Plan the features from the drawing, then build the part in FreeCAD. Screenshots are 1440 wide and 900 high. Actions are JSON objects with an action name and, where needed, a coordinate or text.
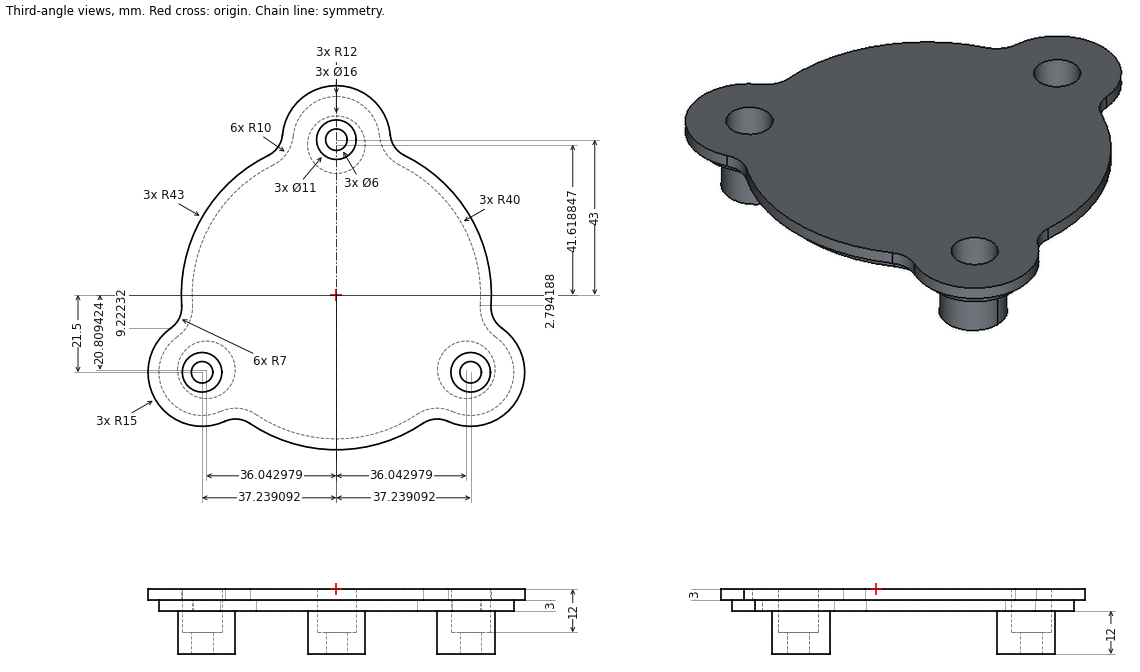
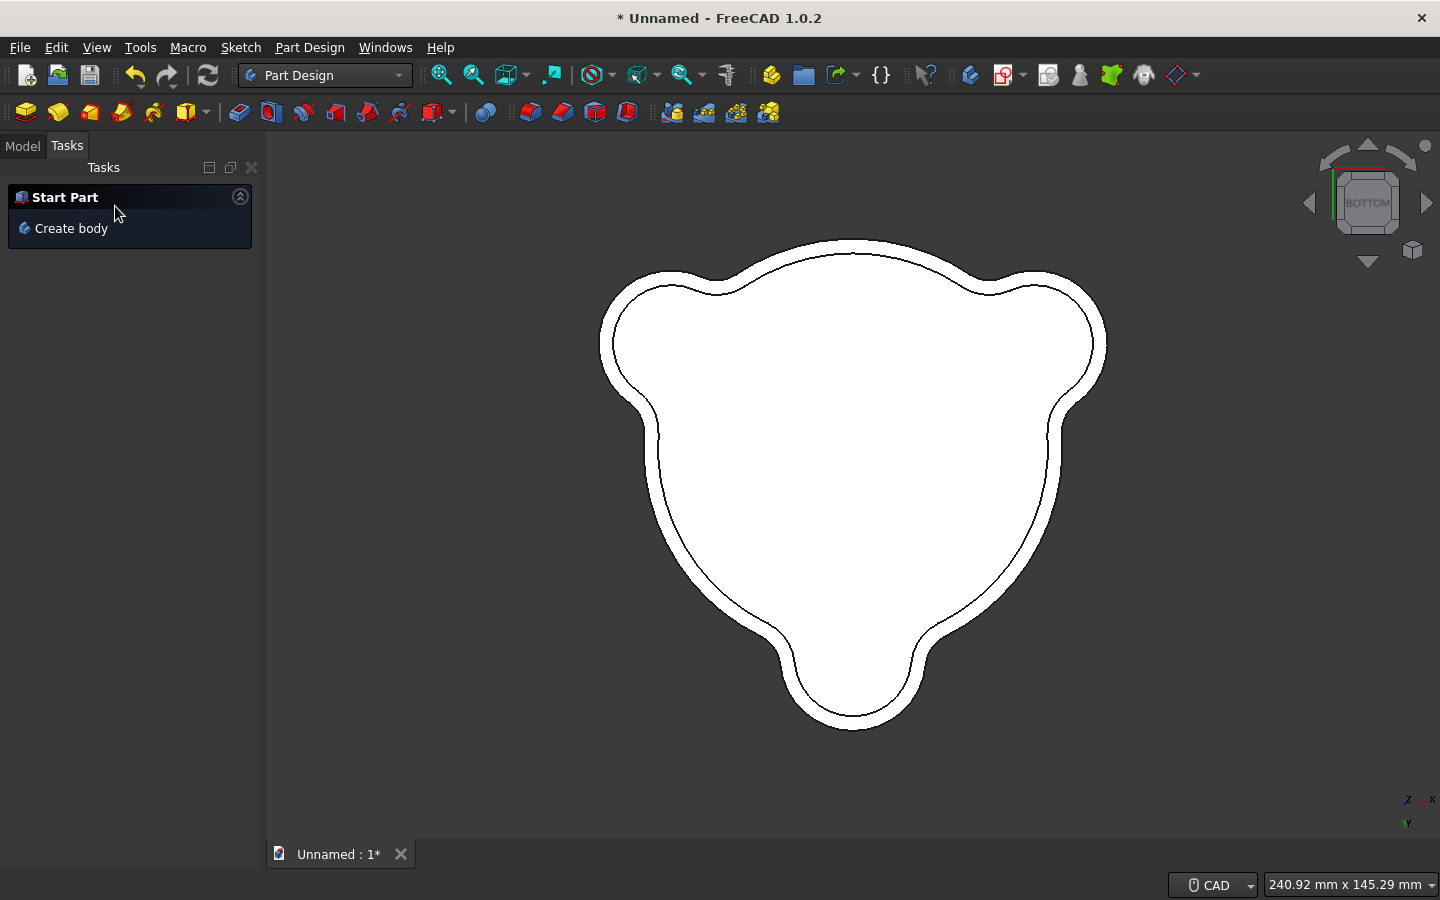
{"action": "left_click", "coordinate": [853, 418]}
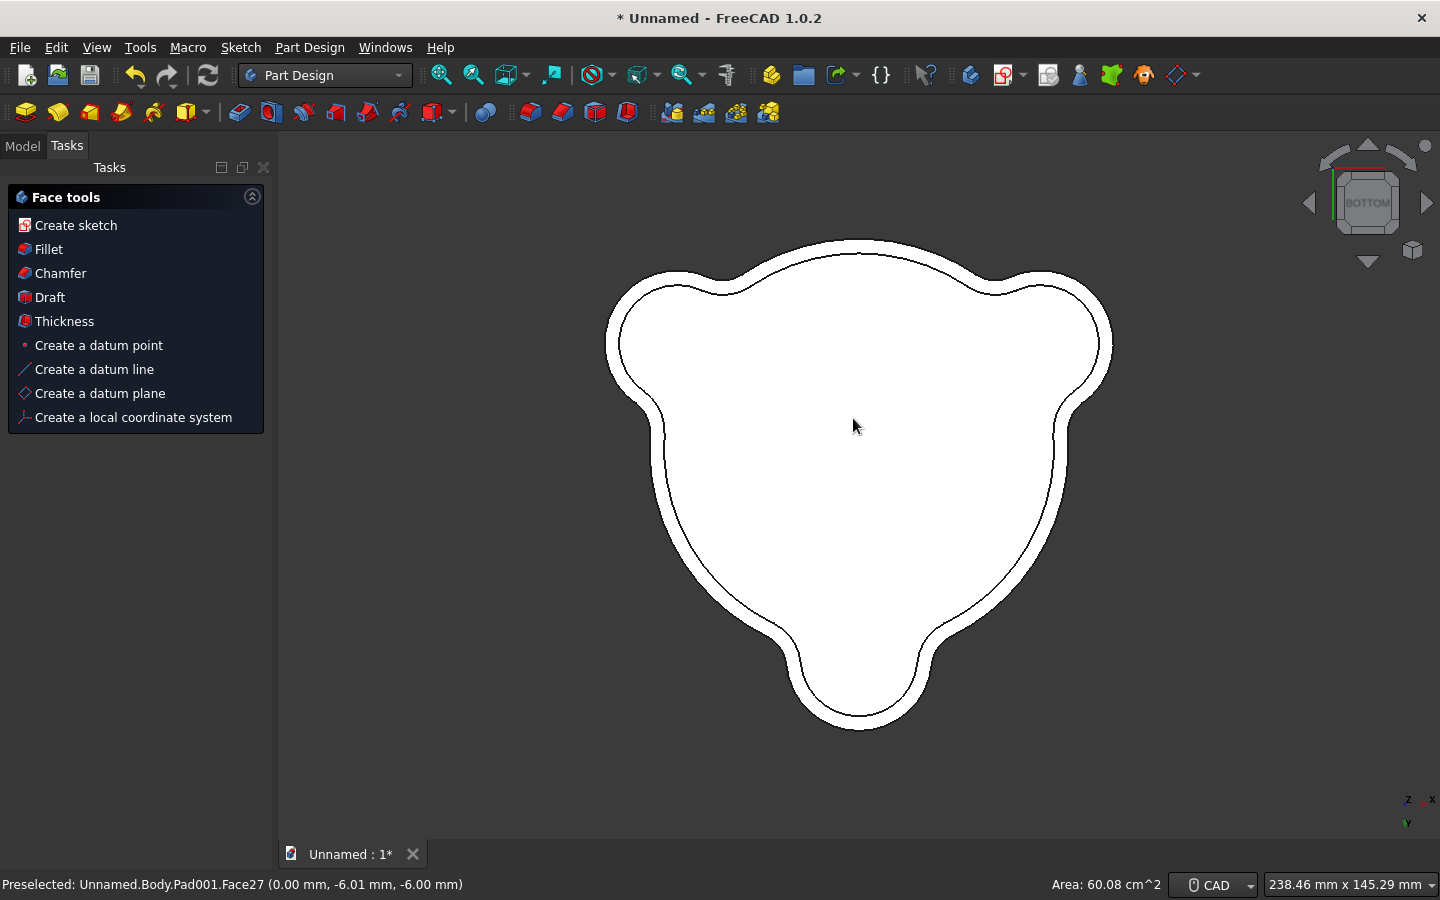
{"action": "left_click", "coordinate": [1004, 76]}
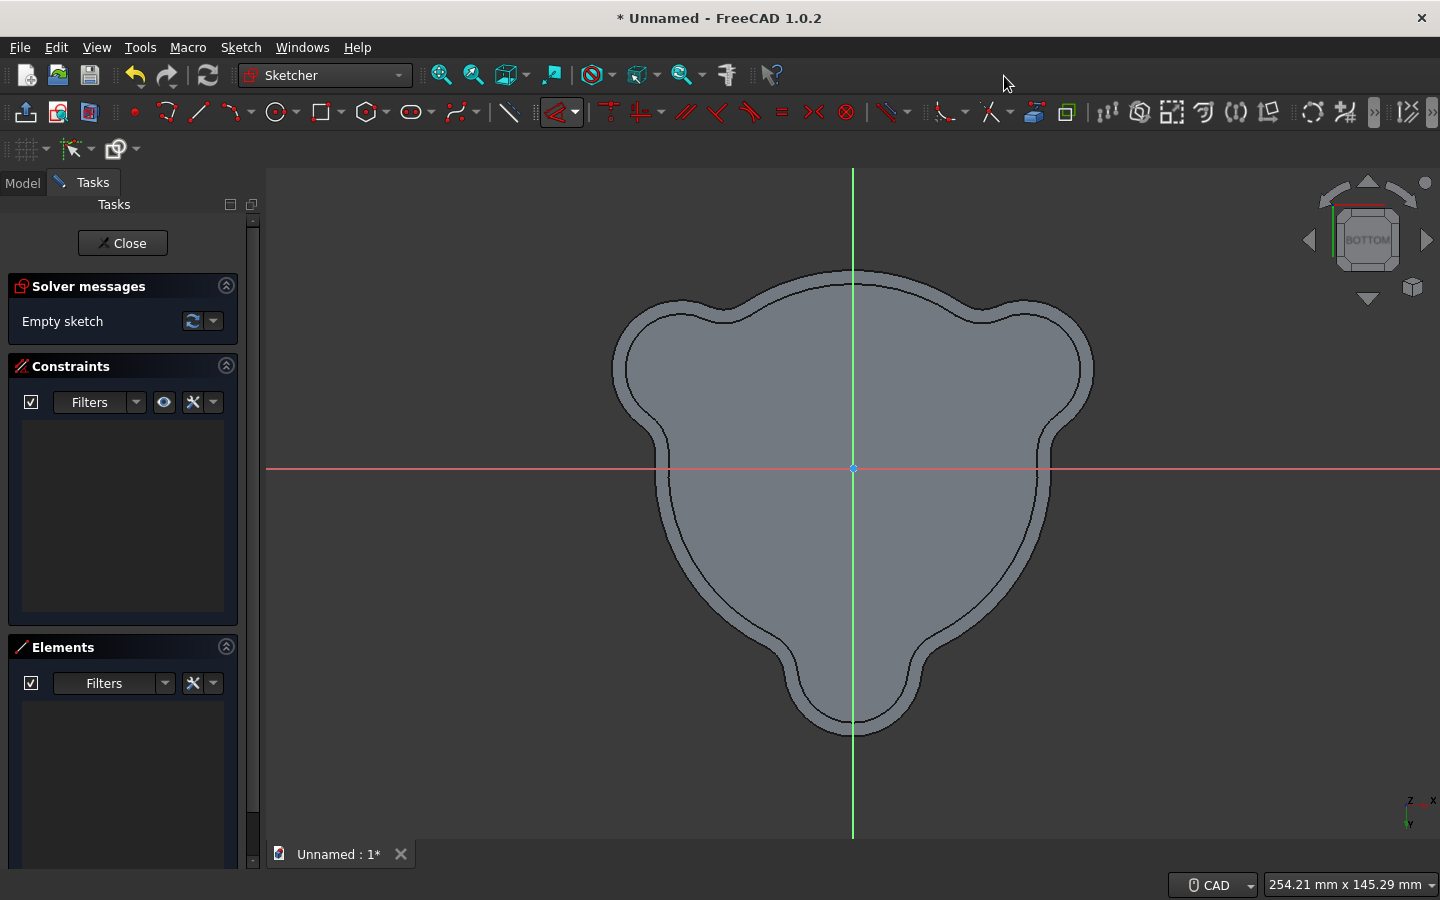
{"action": "left_click", "coordinate": [276, 112]}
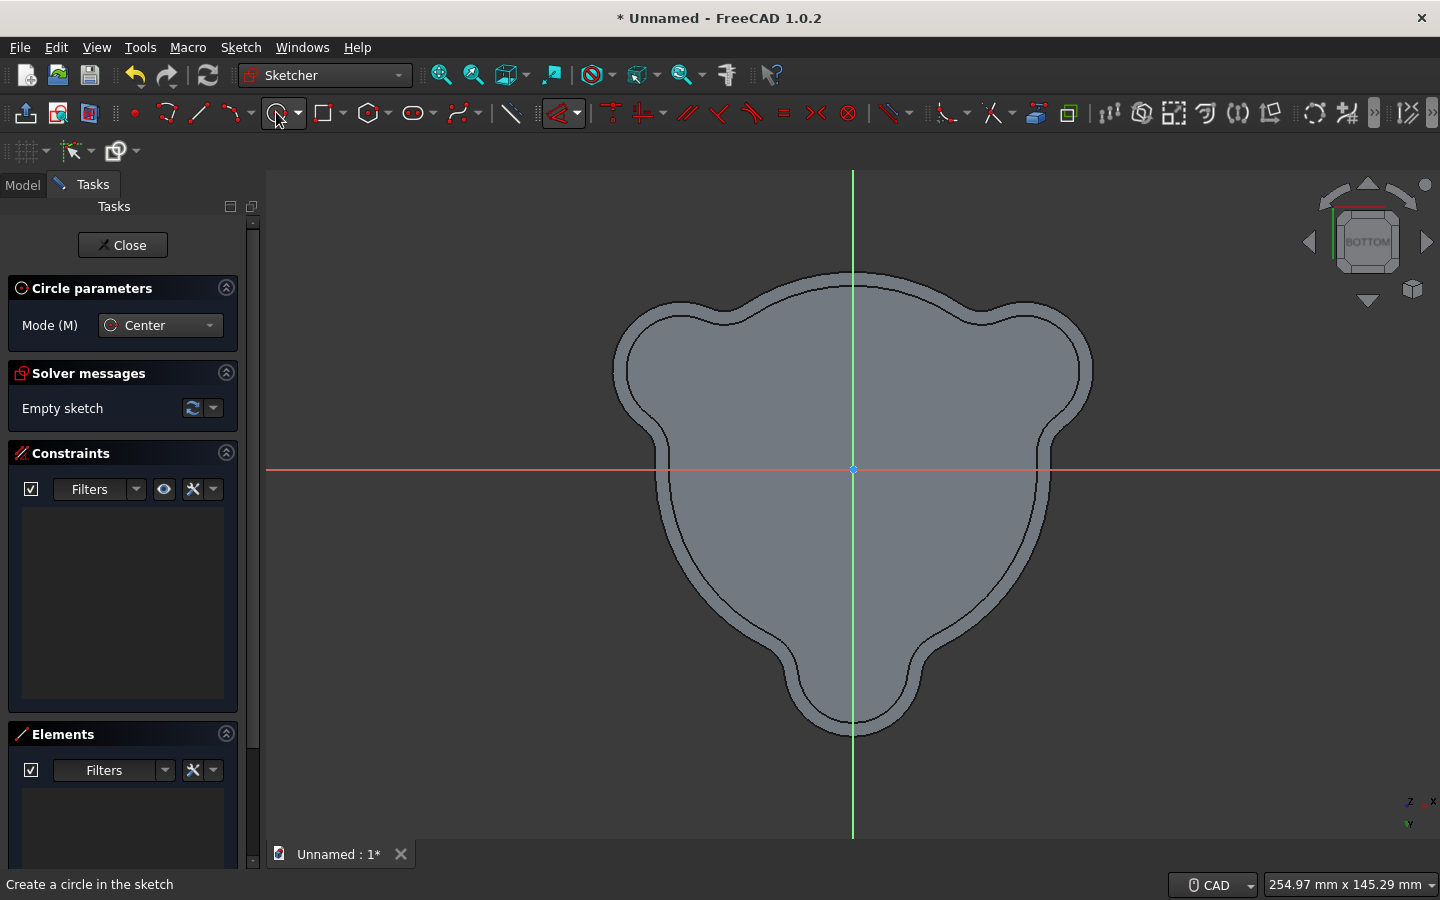
{"action": "left_click", "coordinate": [853, 661]}
{"action": "left_click", "coordinate": [879, 635]}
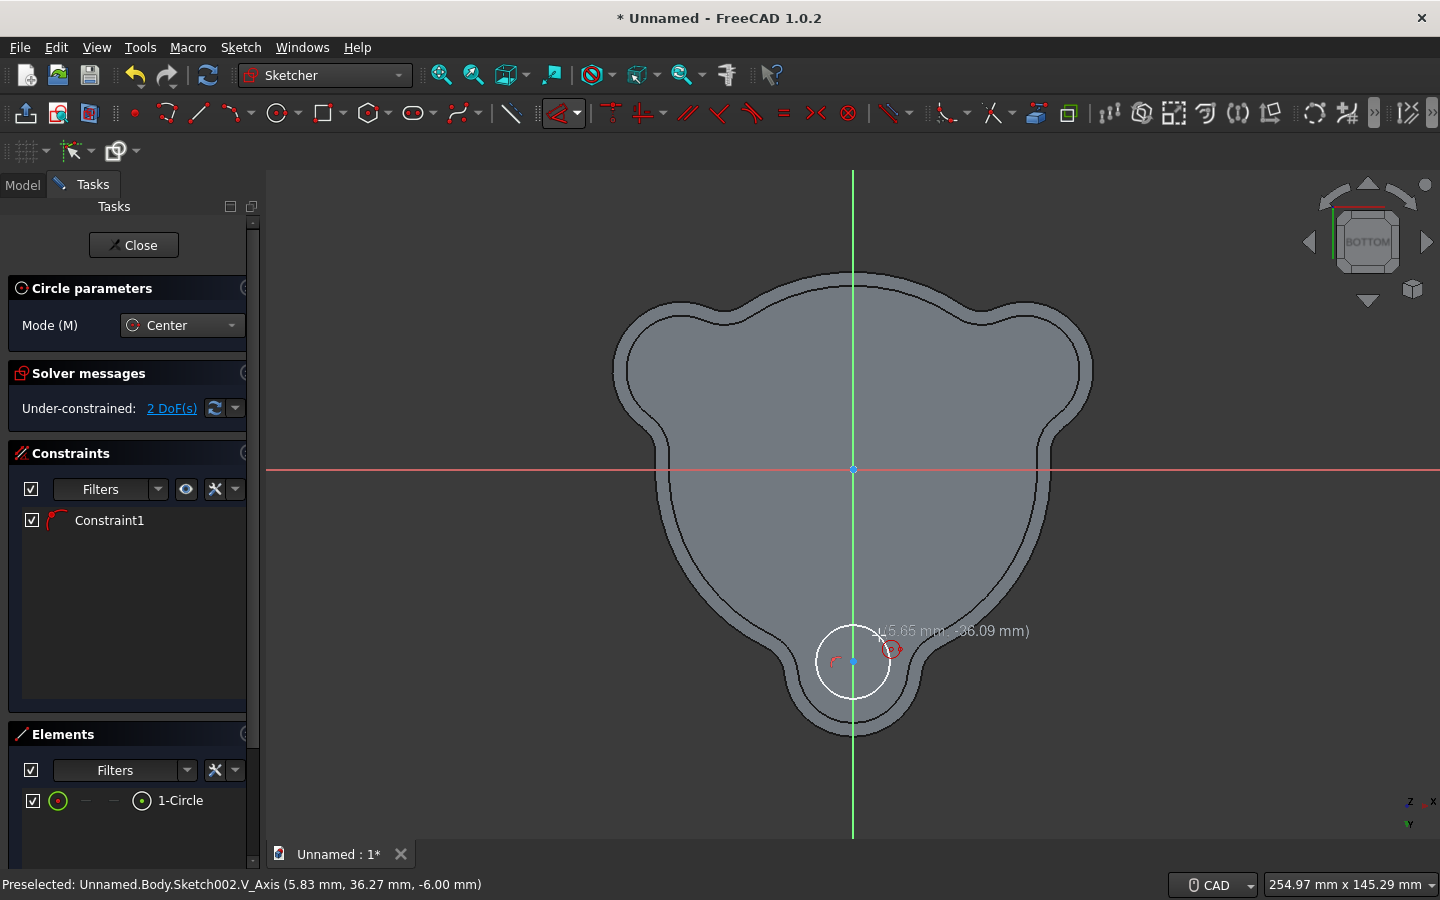
{"action": "left_click", "coordinate": [687, 374]}
{"action": "left_click", "coordinate": [713, 348]}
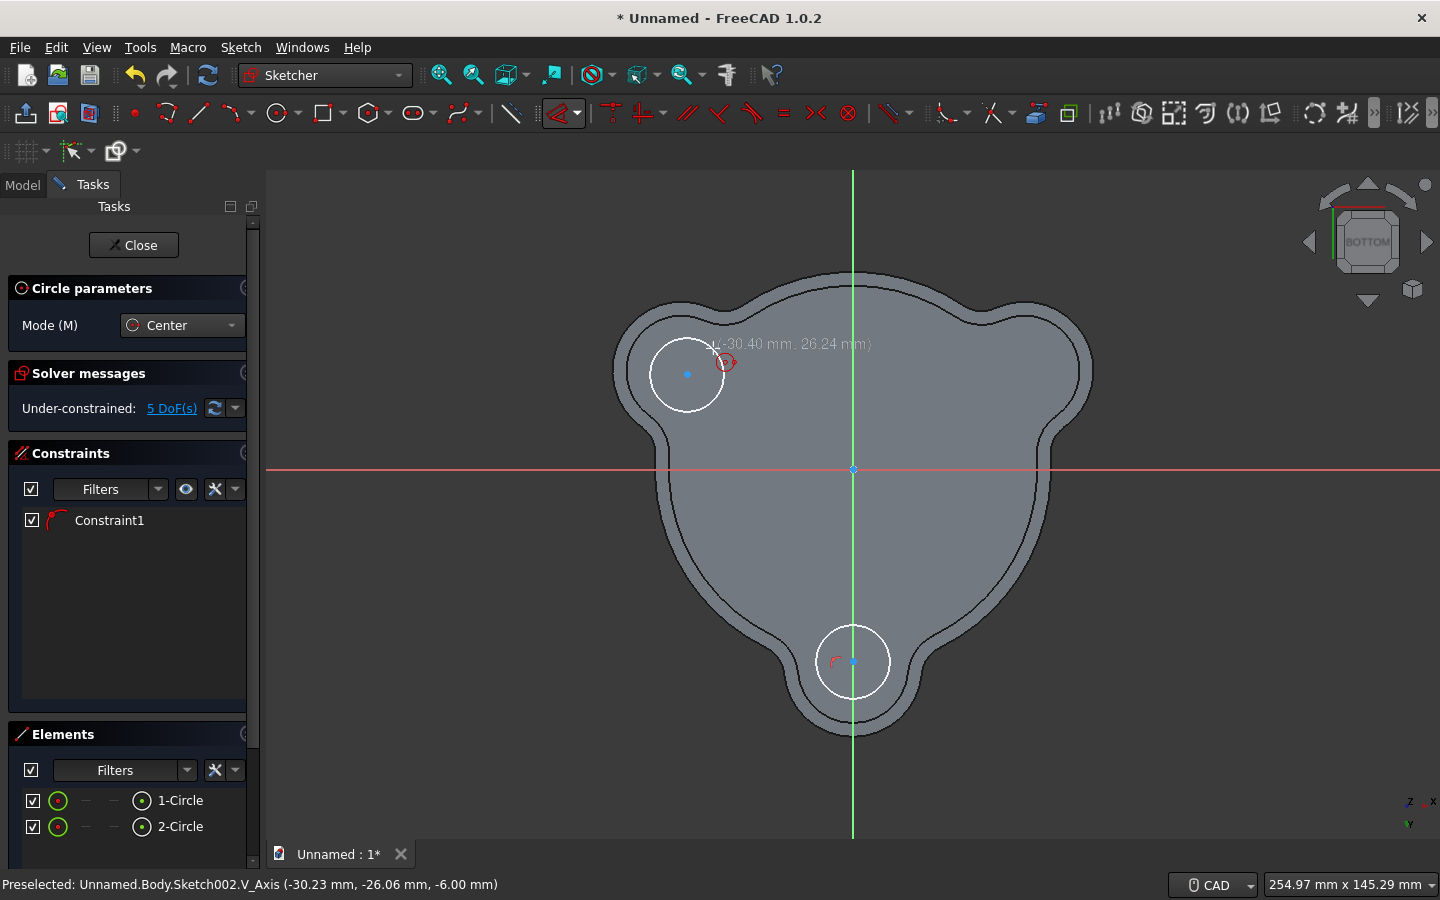
{"action": "left_click", "coordinate": [1019, 374]}
{"action": "left_click", "coordinate": [1045, 348]}
{"action": "key", "text": "Escape"}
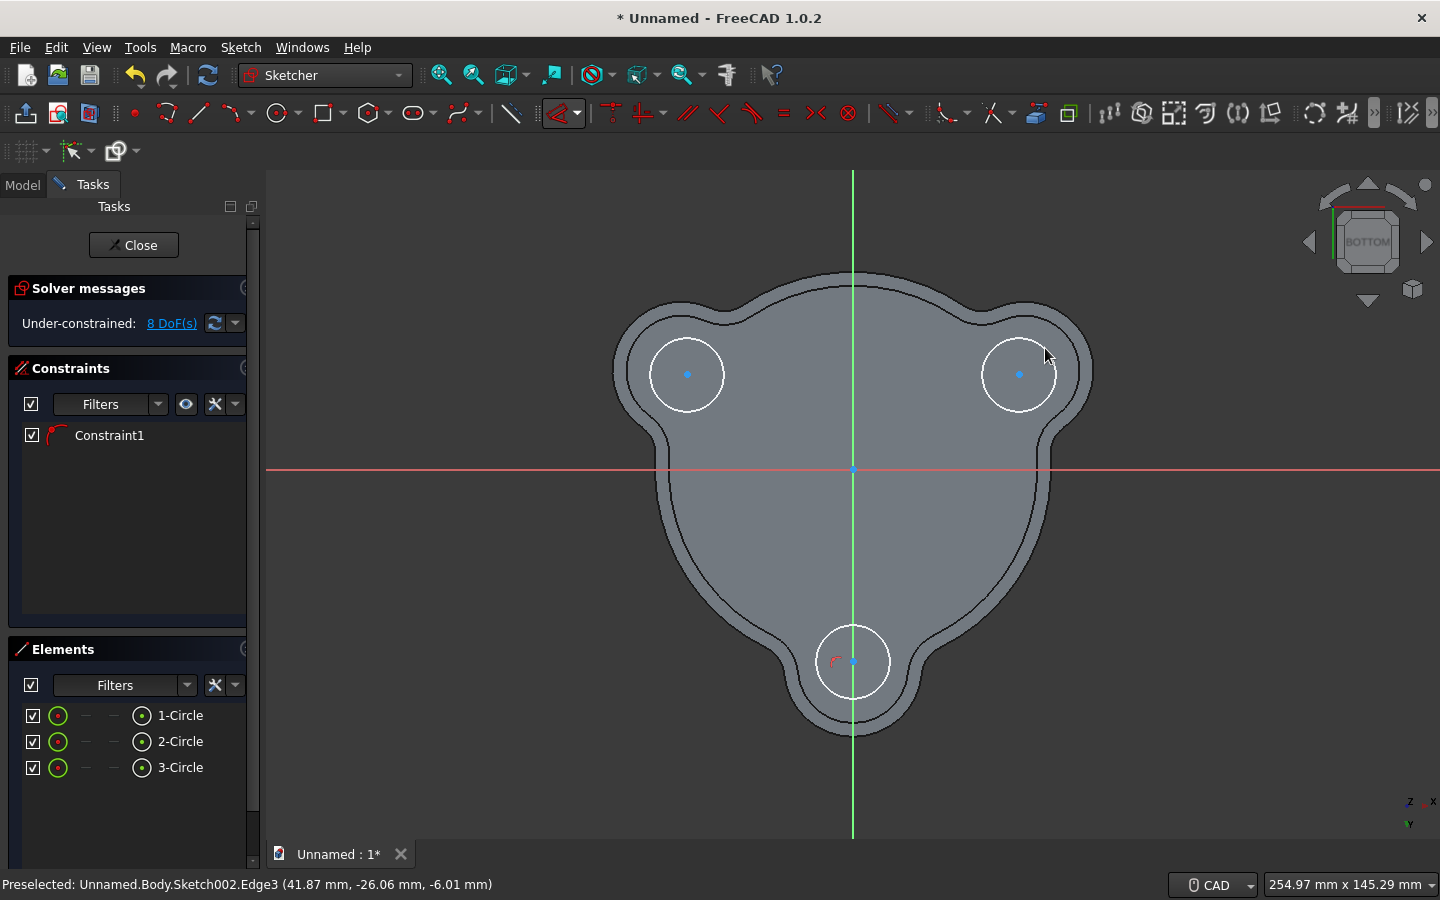
{"action": "left_click", "coordinate": [879, 636]}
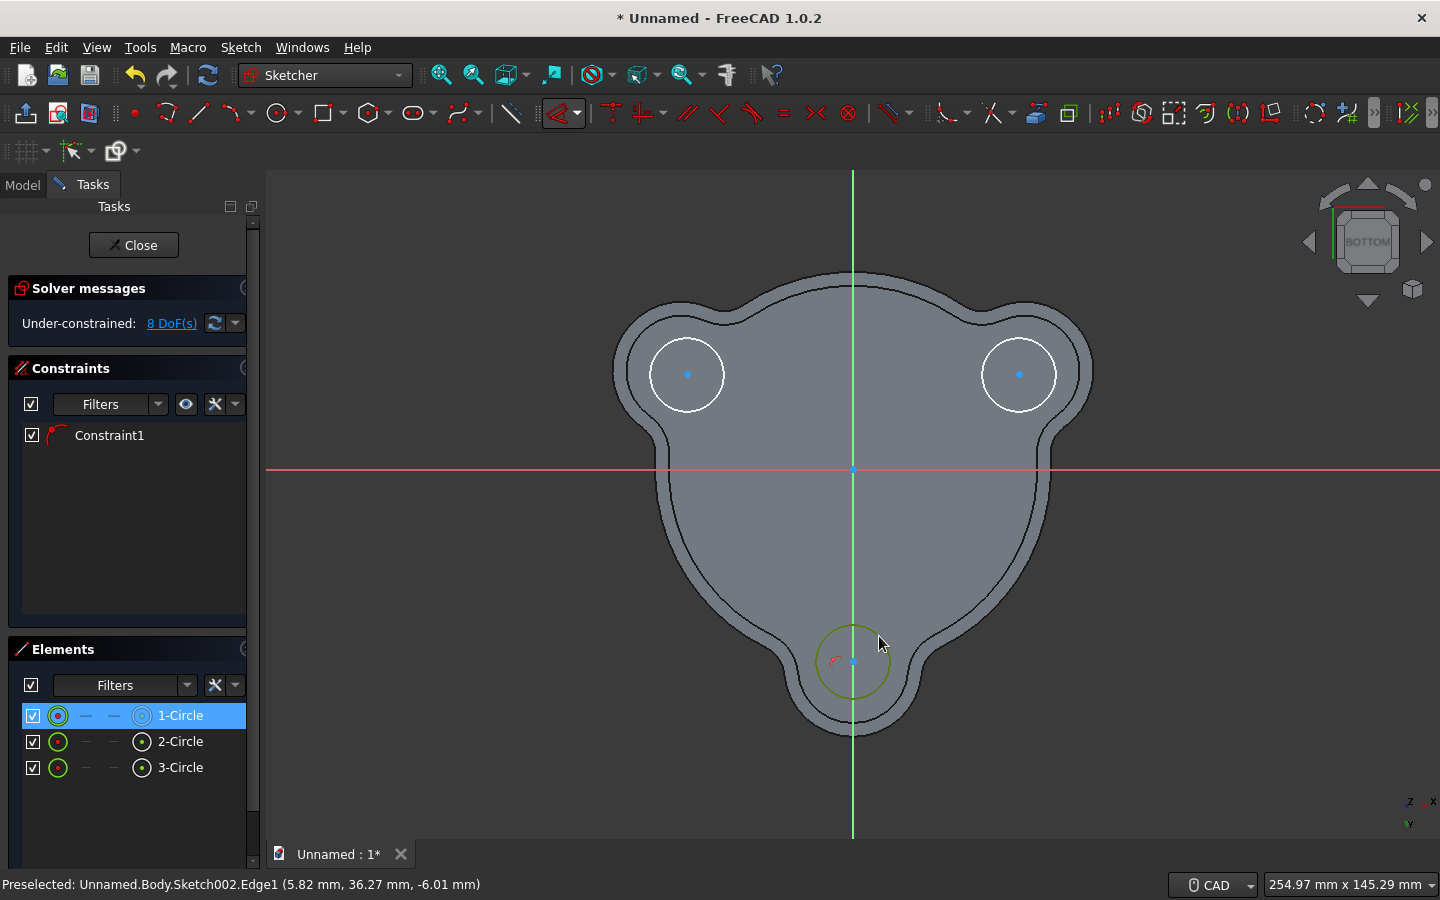
{"action": "left_click", "coordinate": [713, 349]}